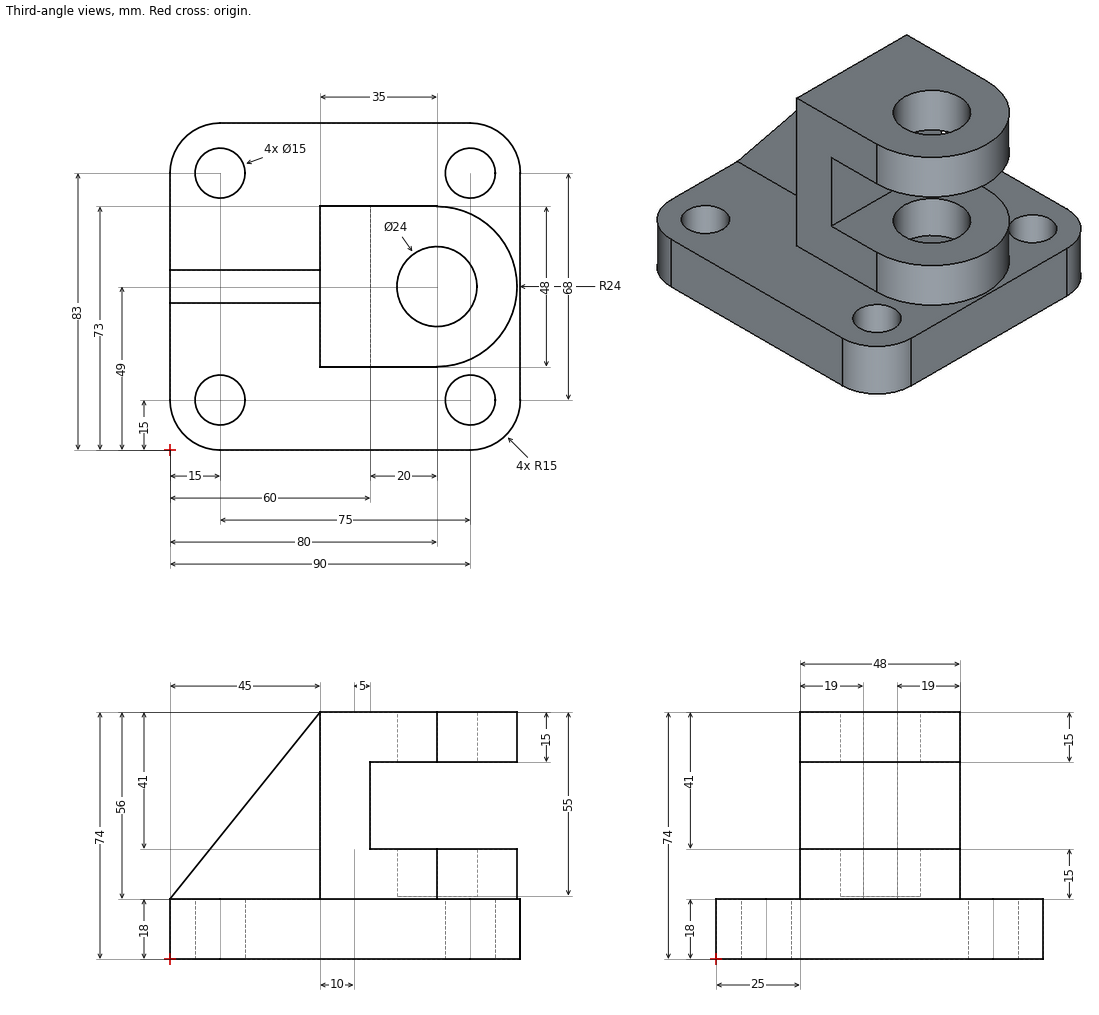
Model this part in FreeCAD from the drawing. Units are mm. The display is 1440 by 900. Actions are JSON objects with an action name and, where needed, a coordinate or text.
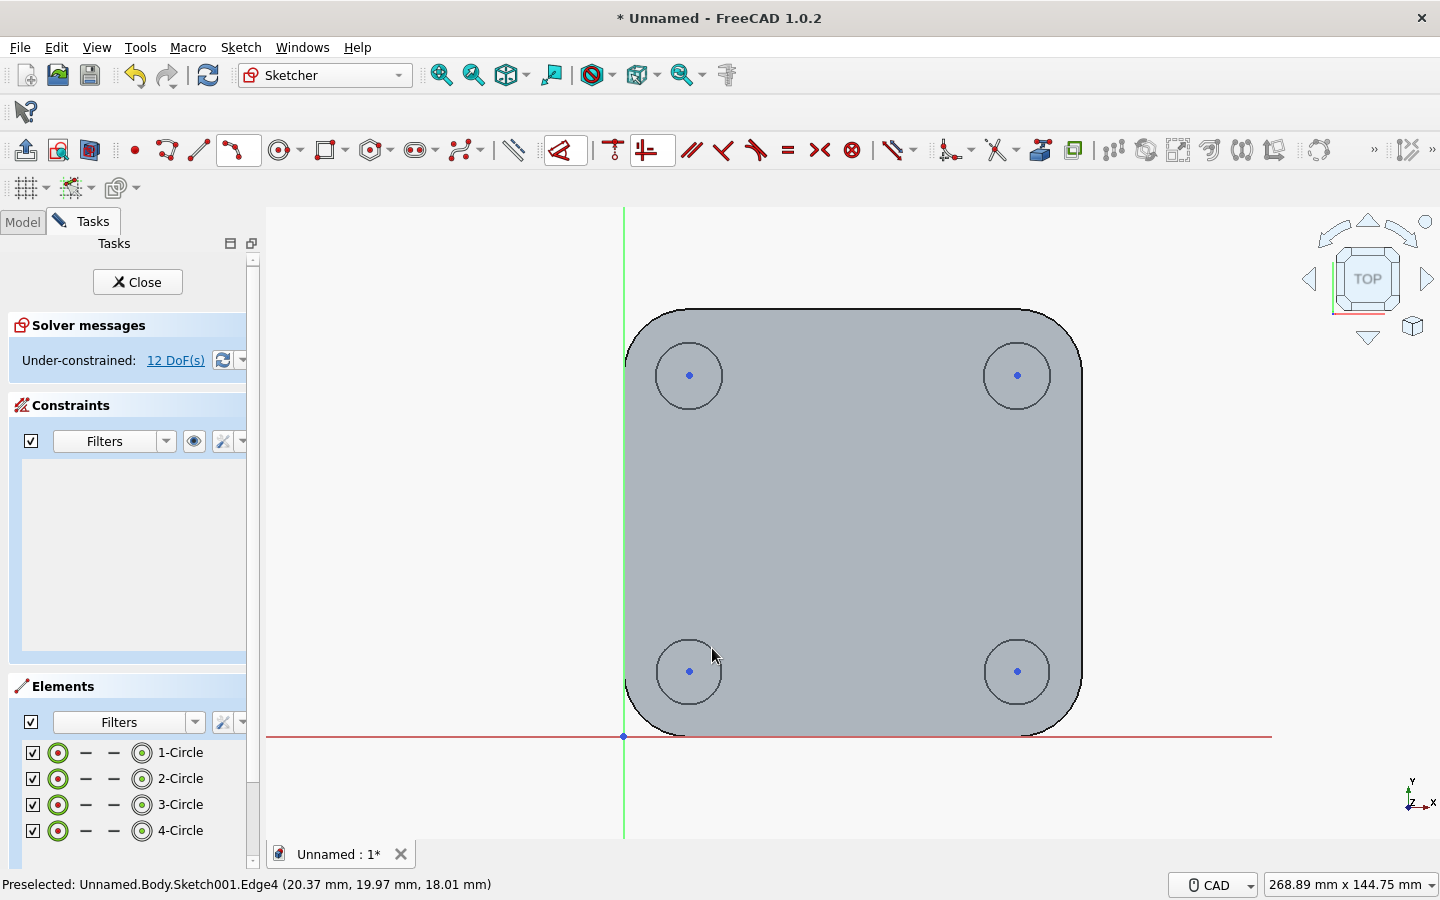
{"action": "left_click", "coordinate": [712, 352]}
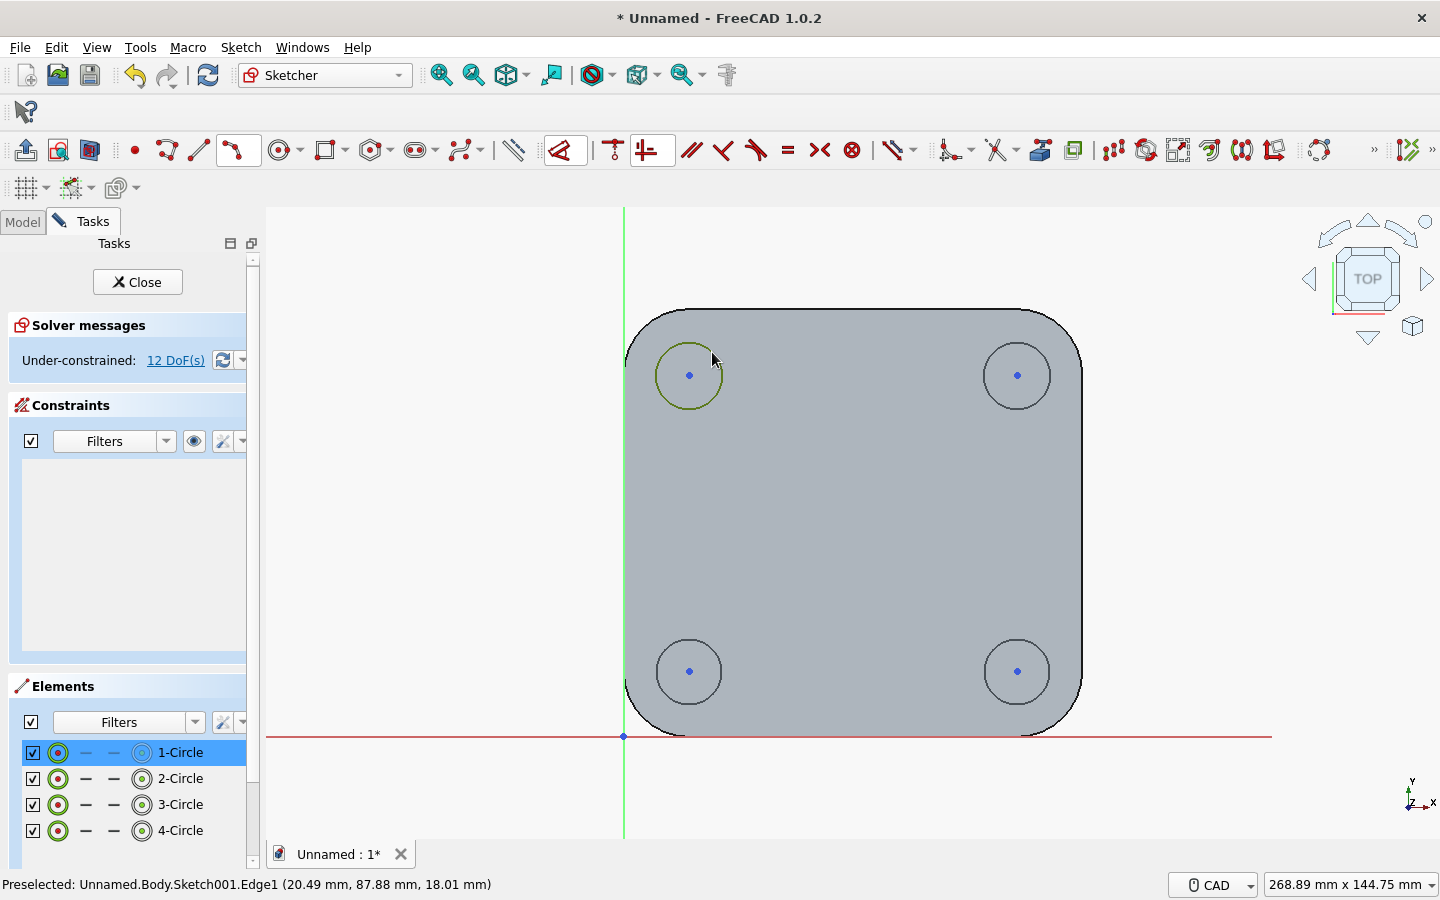
{"action": "left_click", "coordinate": [1040, 352]}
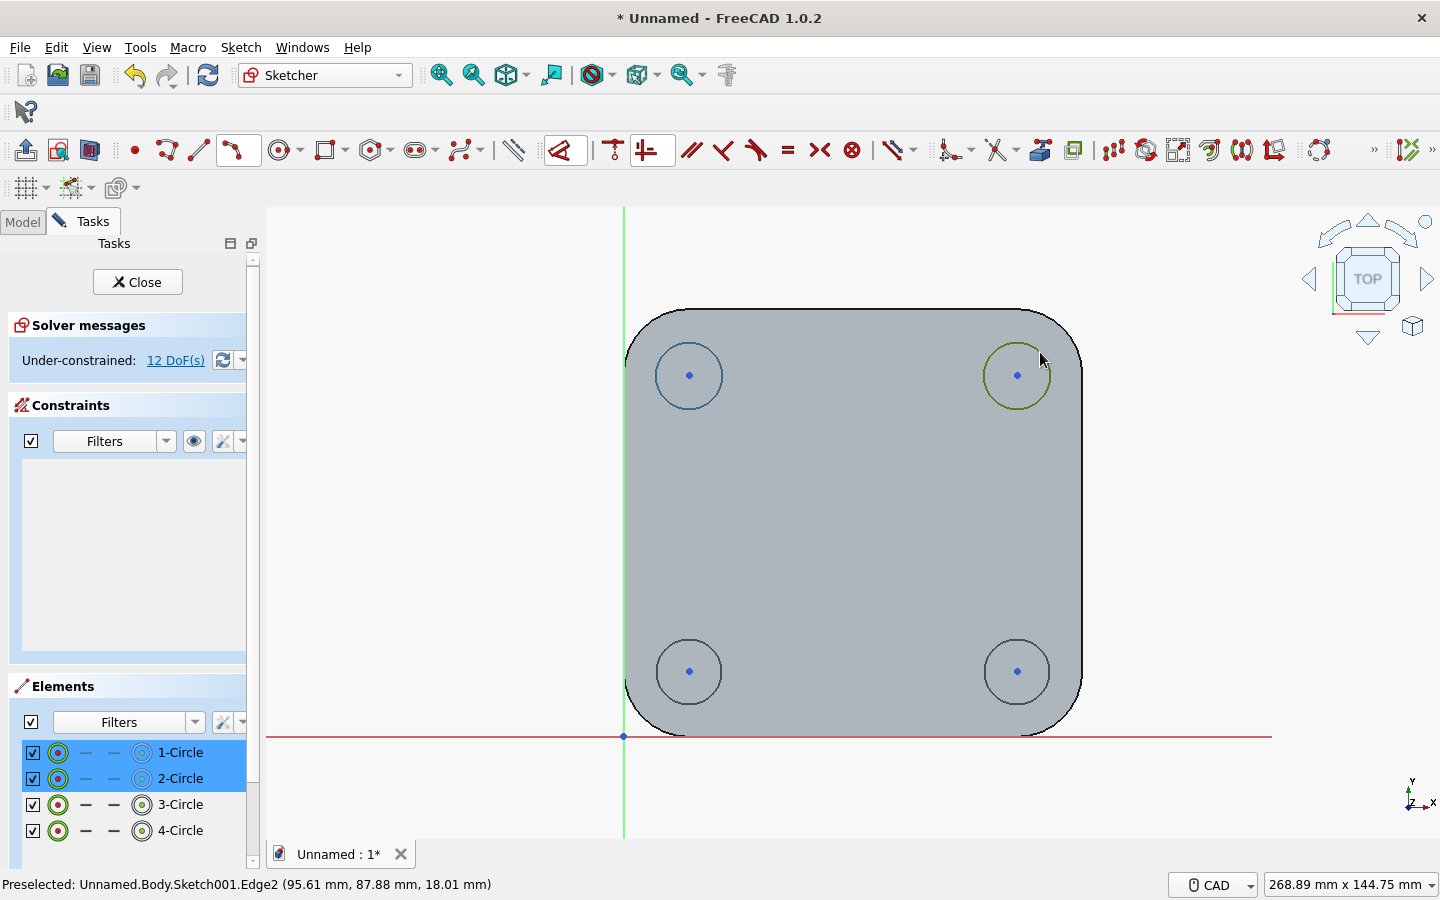
{"action": "left_click", "coordinate": [1040, 649]}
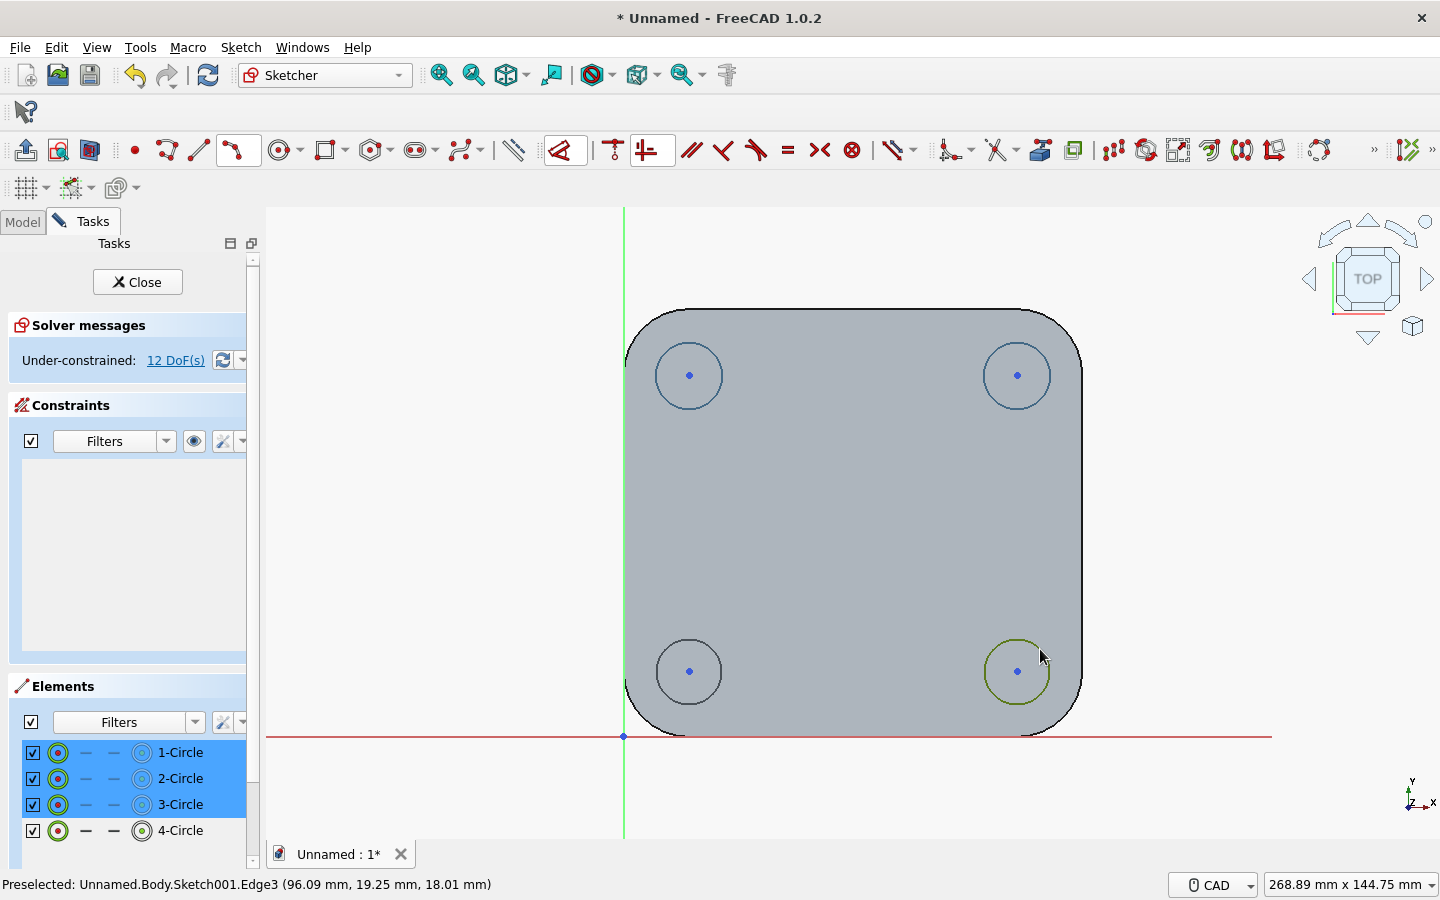
{"action": "left_click", "coordinate": [712, 649]}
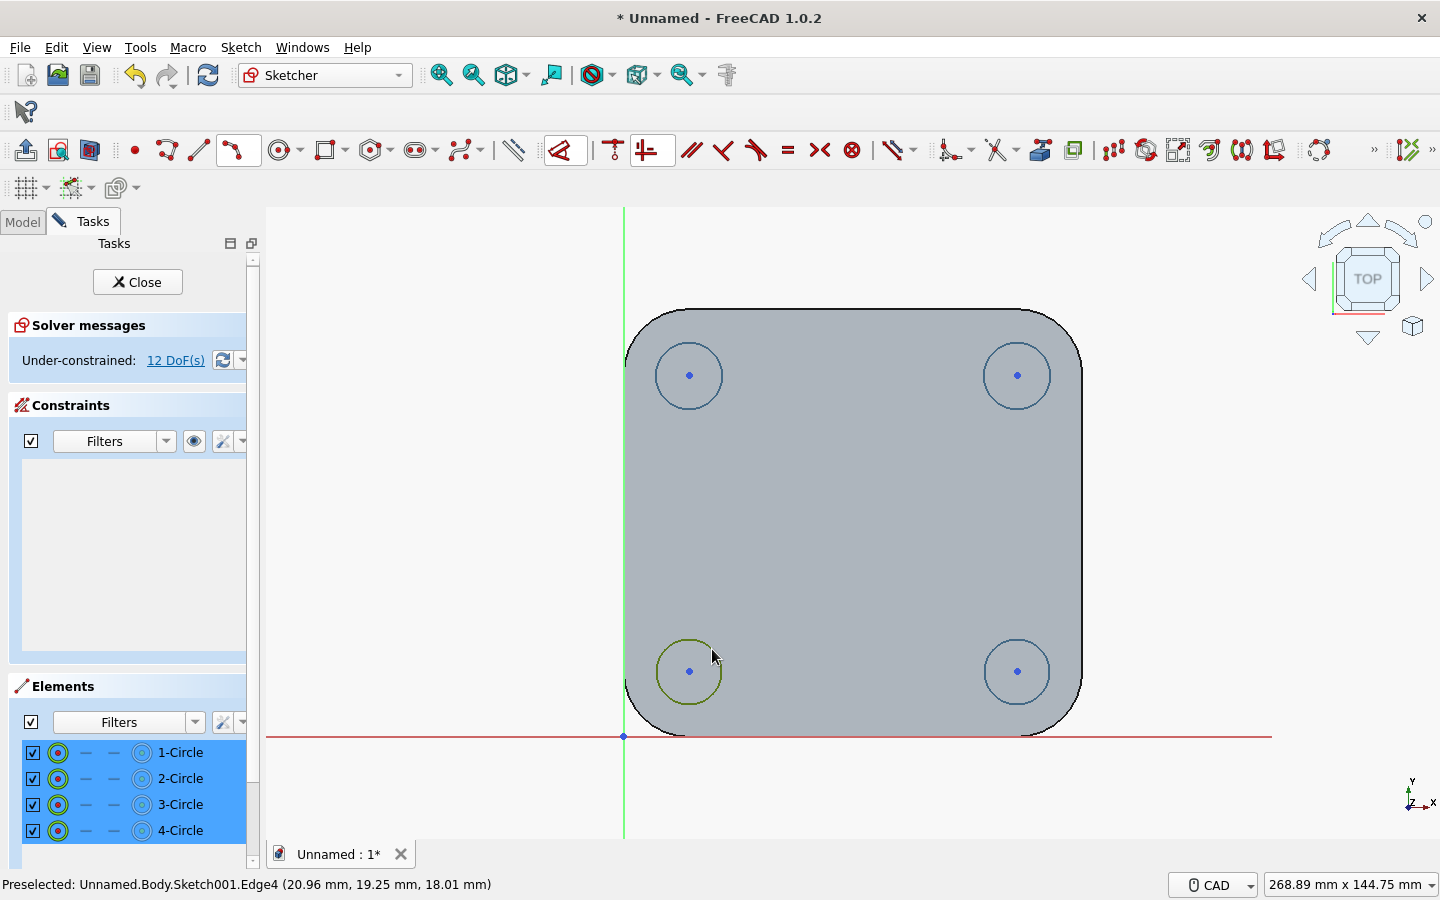
{"action": "left_click", "coordinate": [788, 150]}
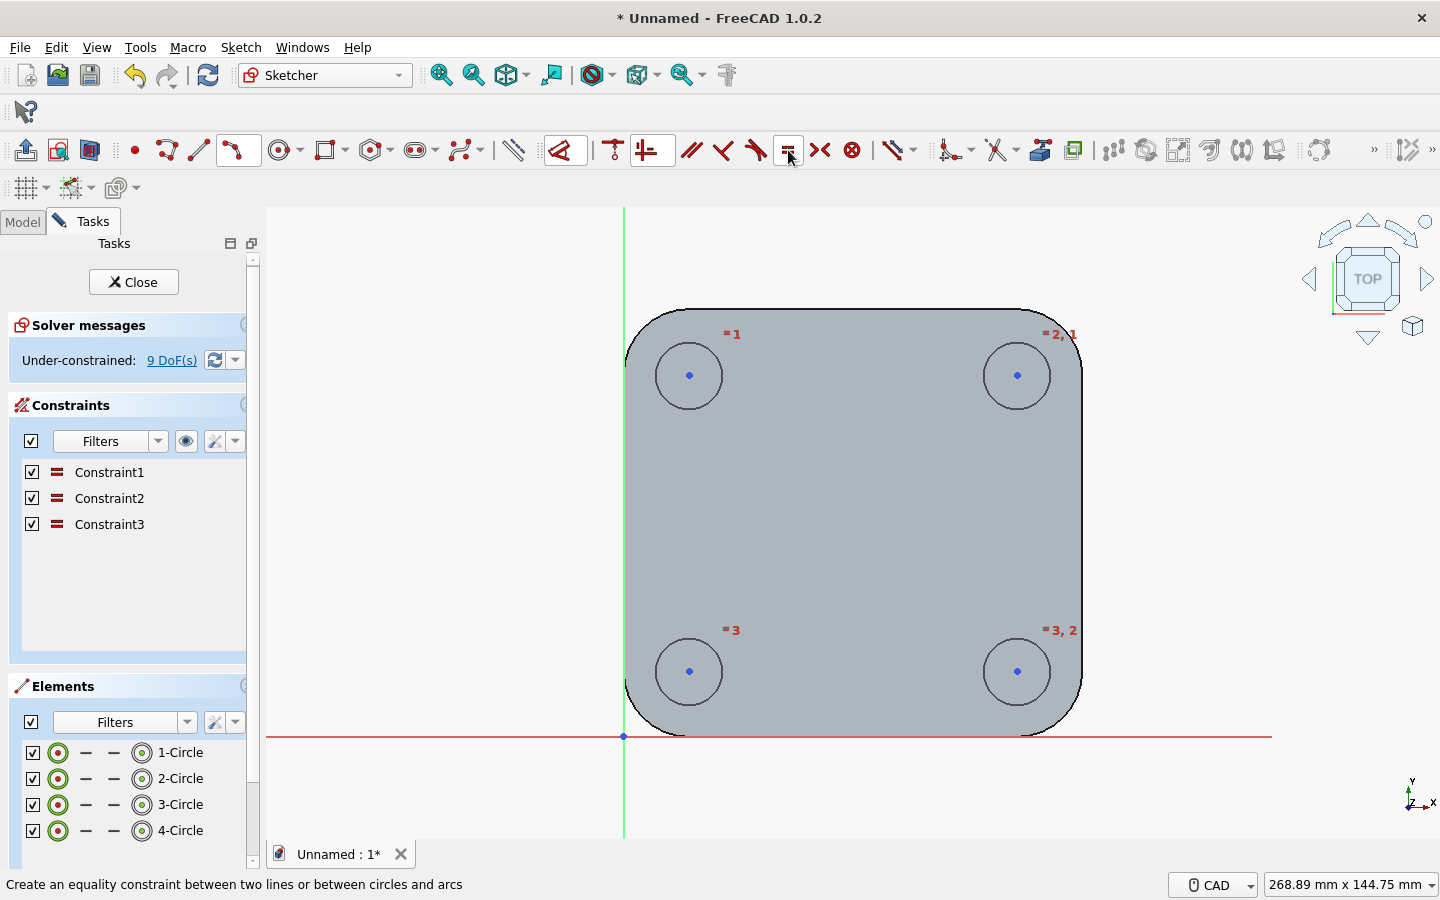
{"action": "left_click", "coordinate": [689, 376]}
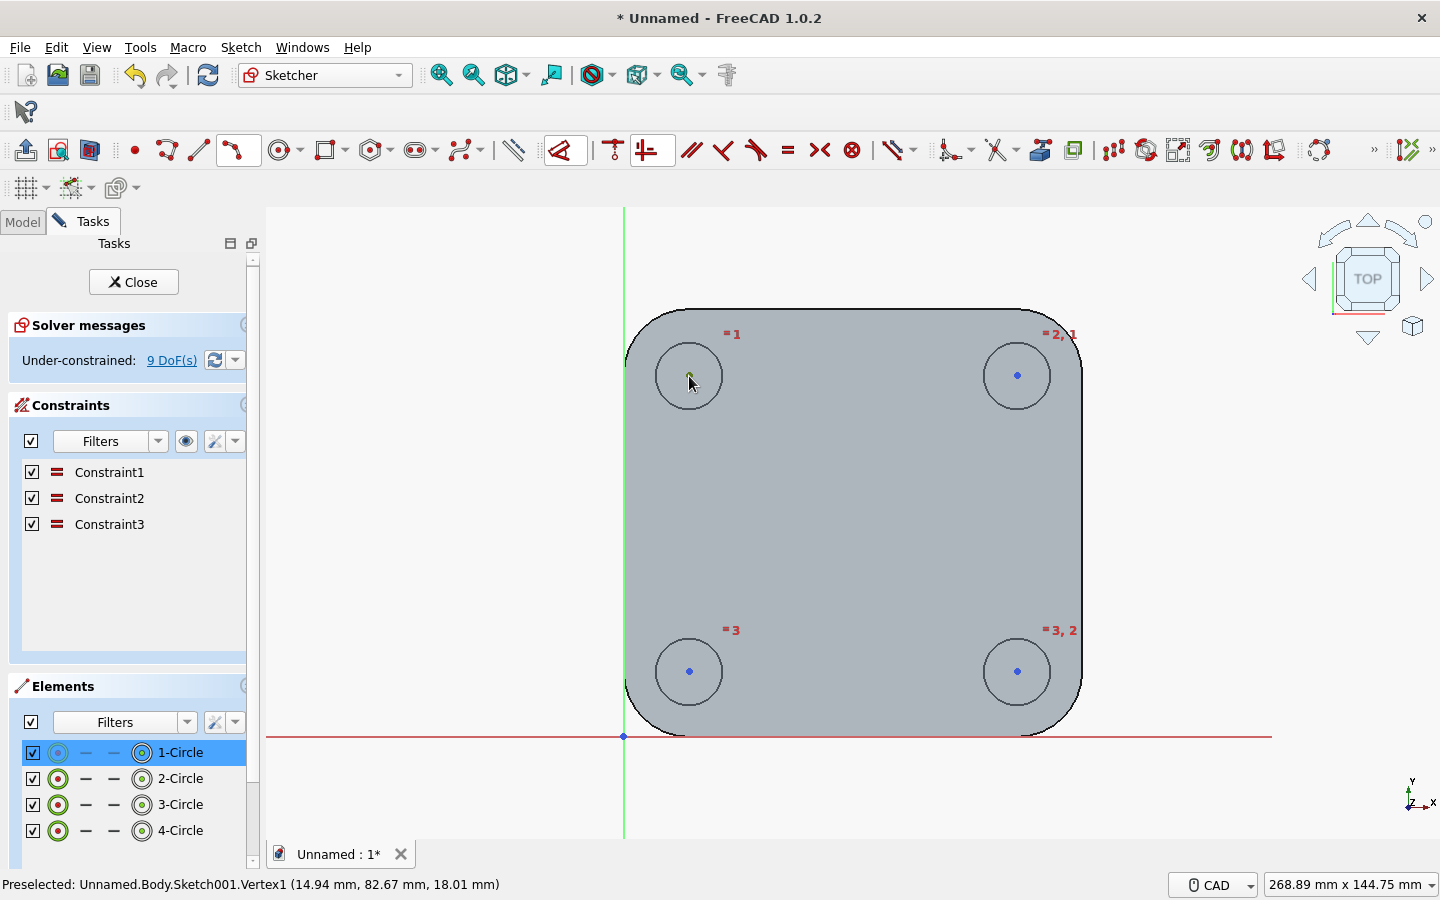
{"action": "left_click", "coordinate": [1017, 376]}